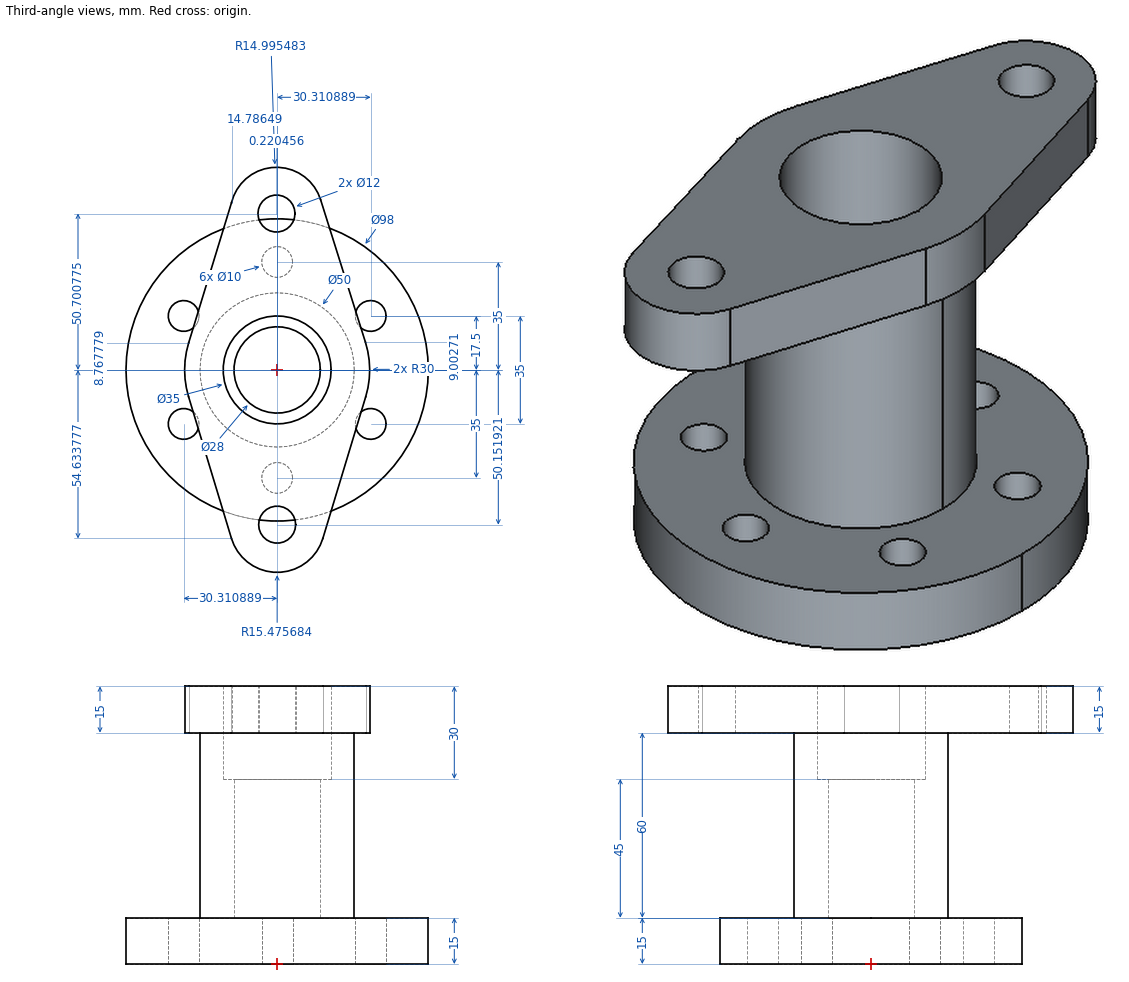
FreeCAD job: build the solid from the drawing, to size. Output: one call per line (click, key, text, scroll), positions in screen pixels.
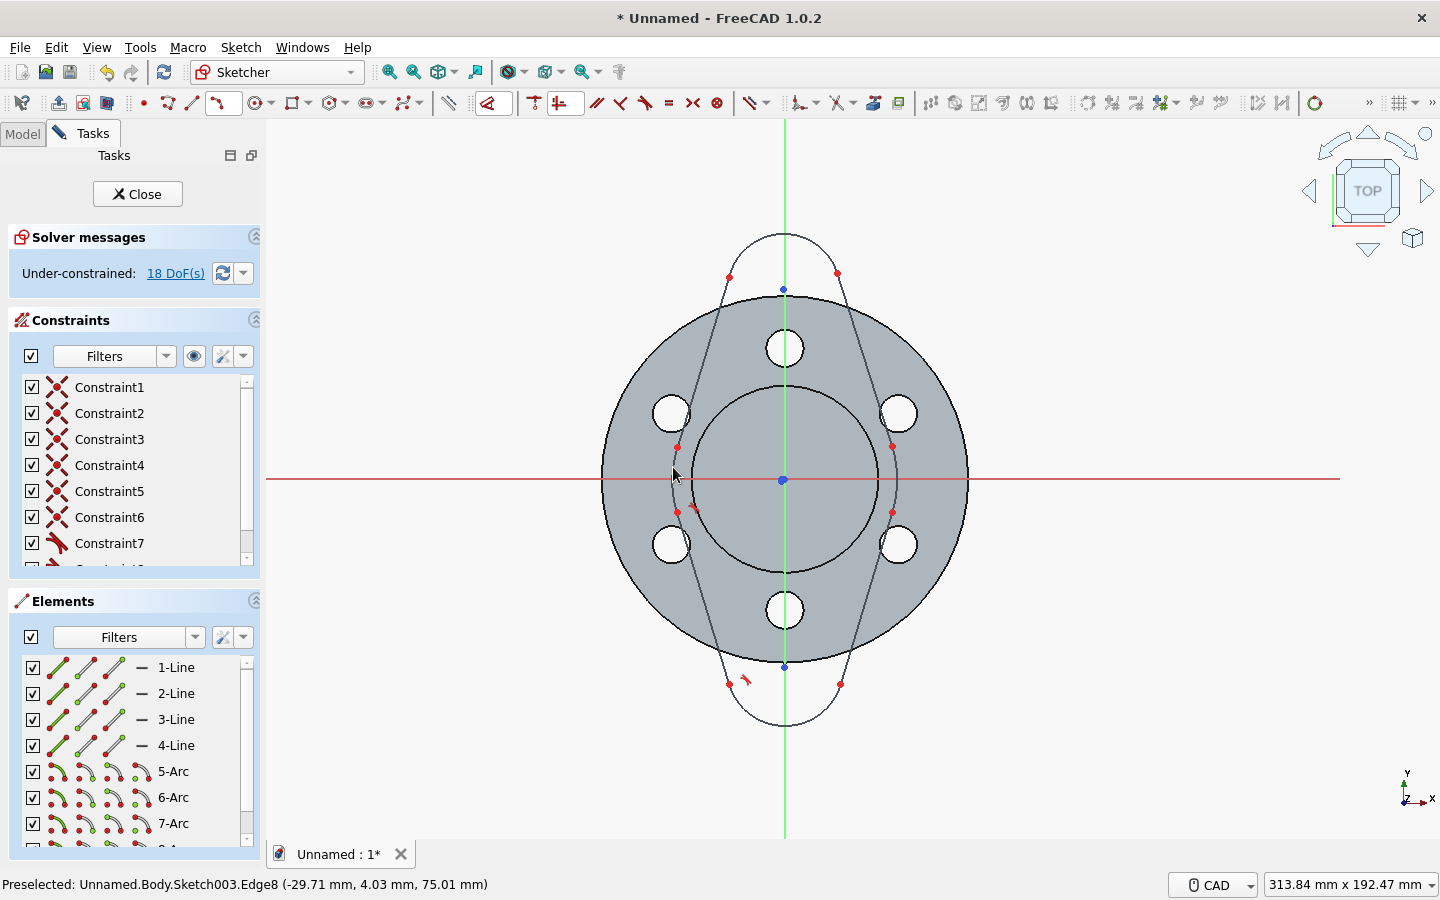
click(856, 633)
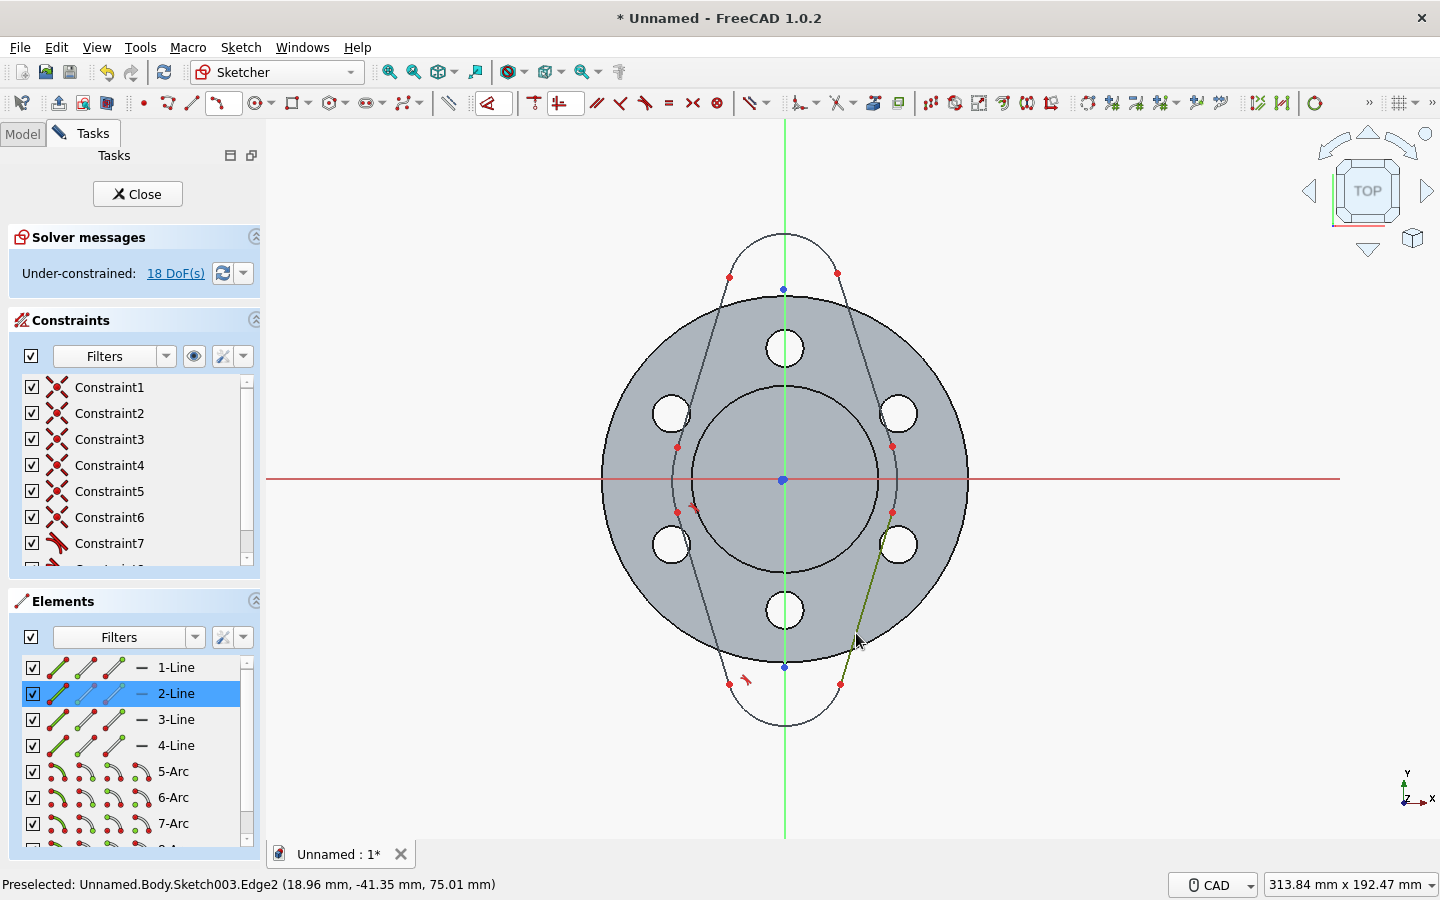
click(757, 719)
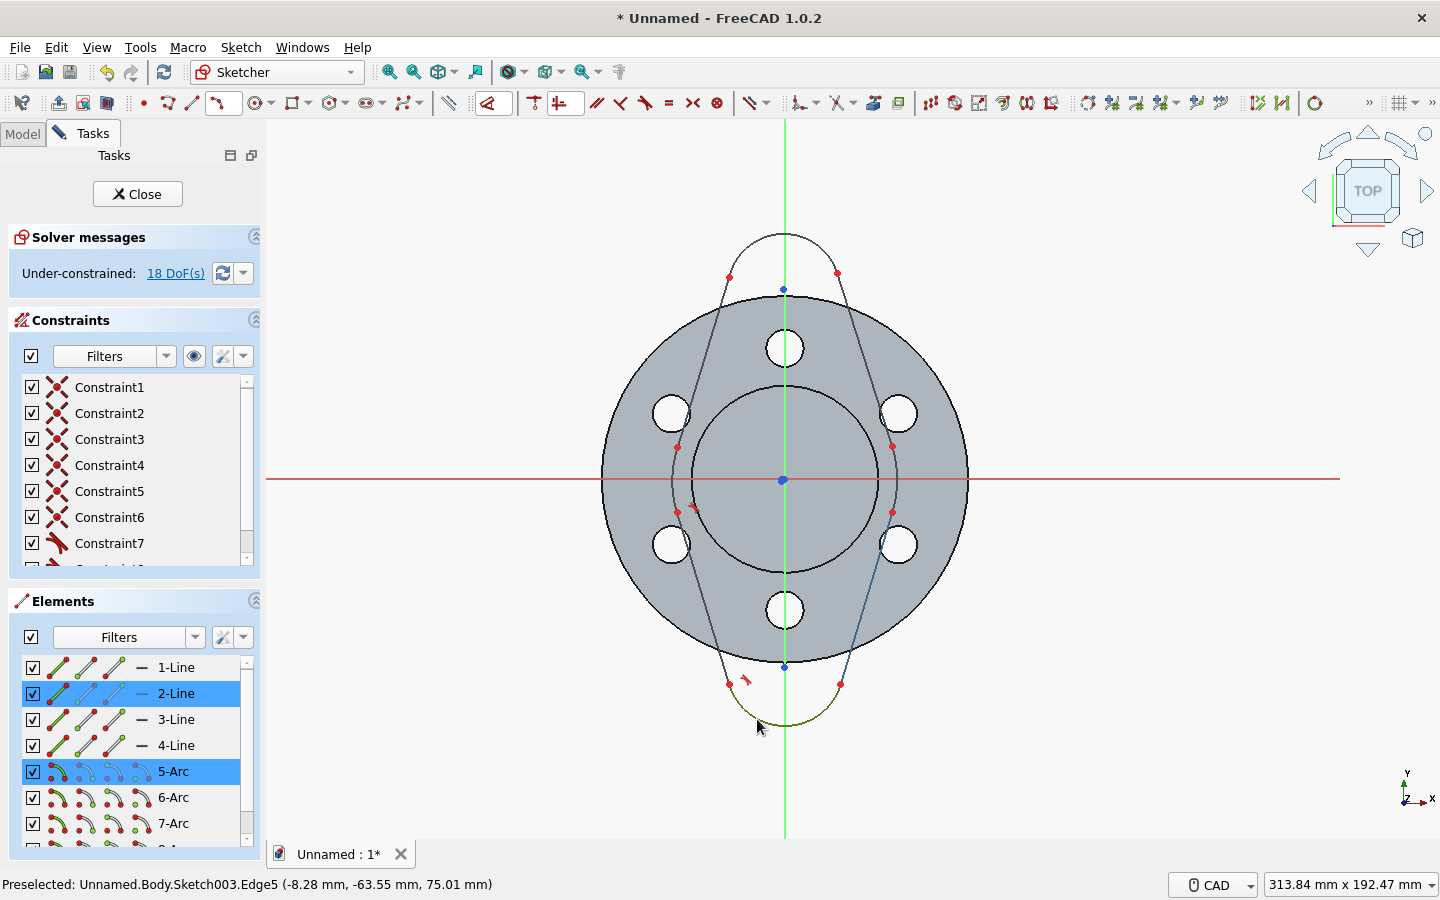
click(646, 104)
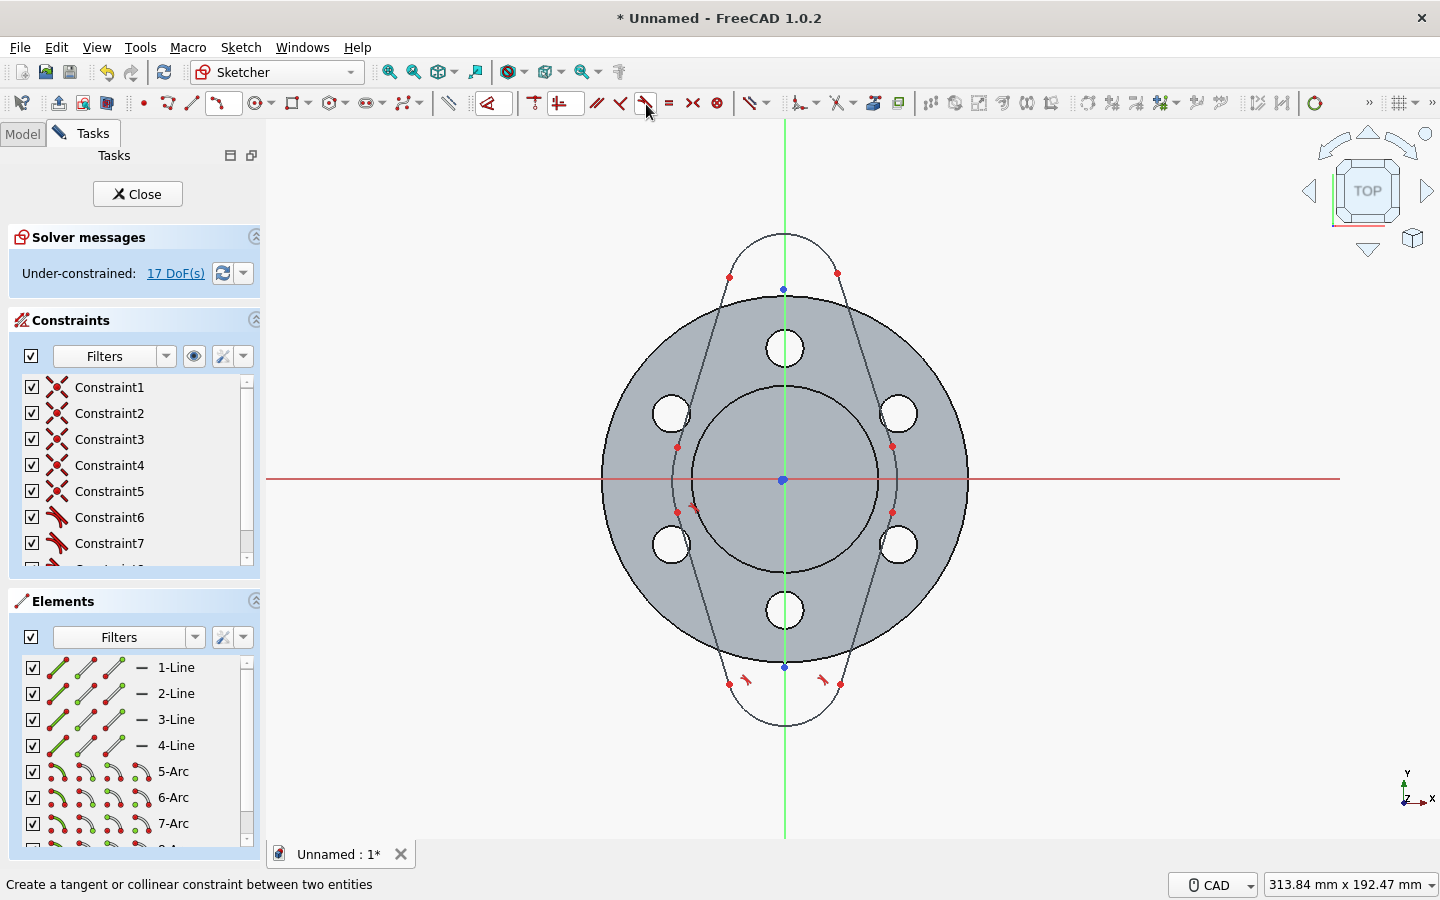
click(856, 633)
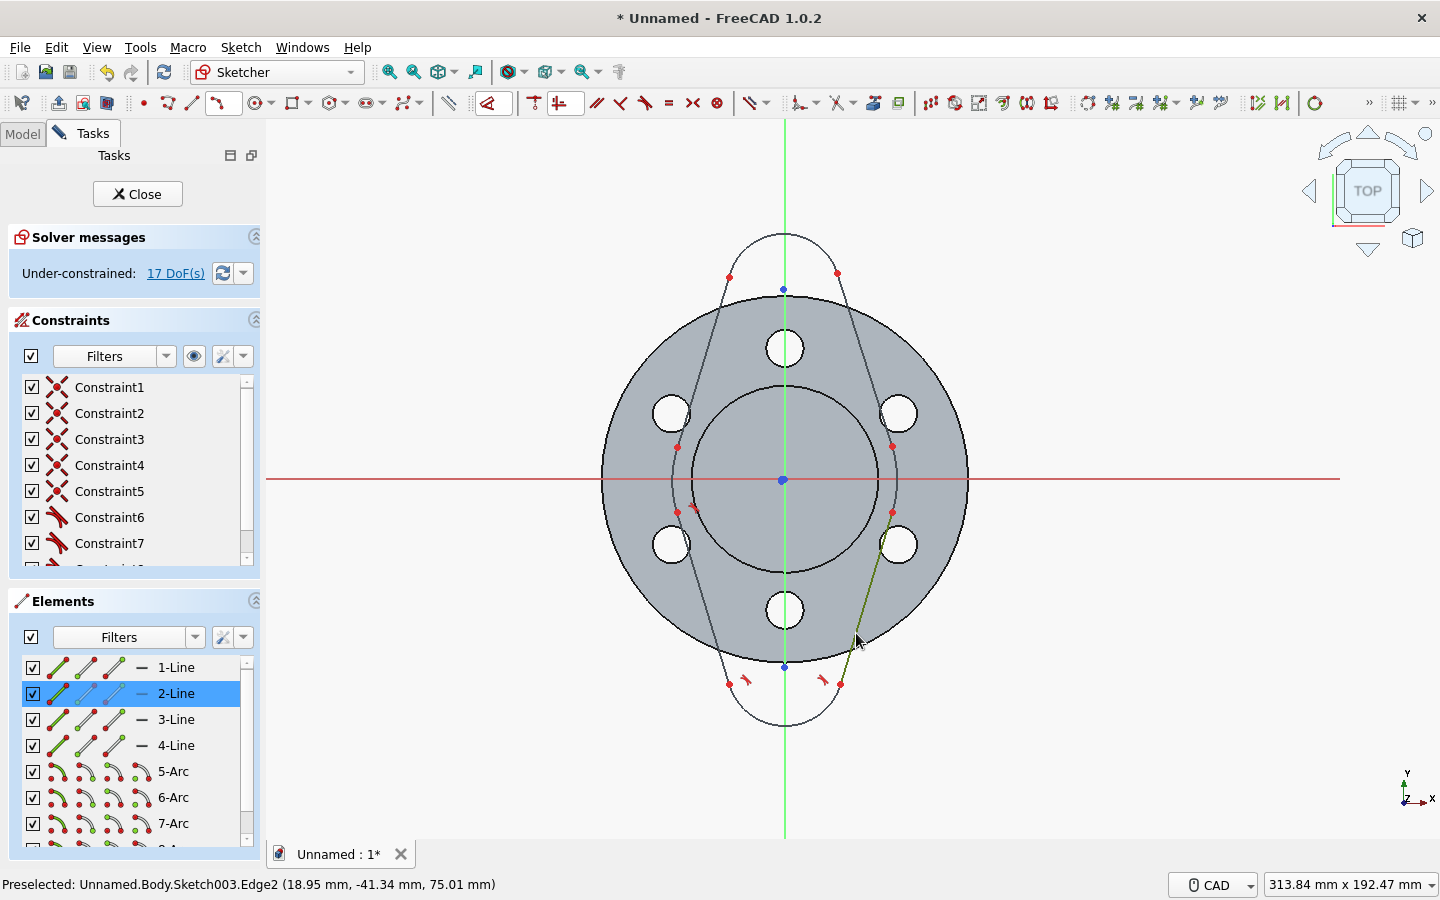
click(896, 493)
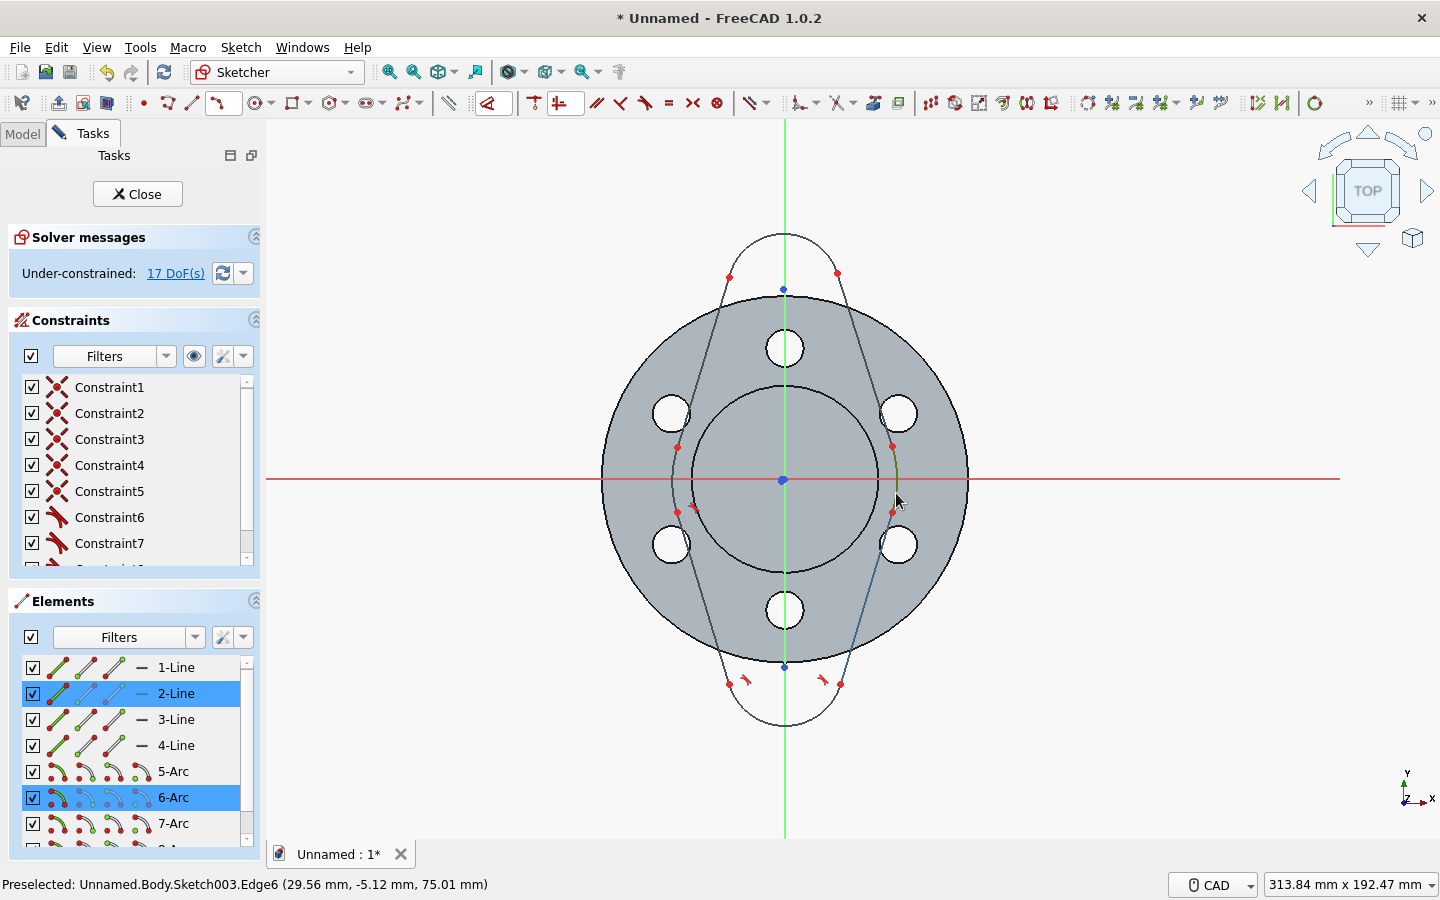
click(646, 104)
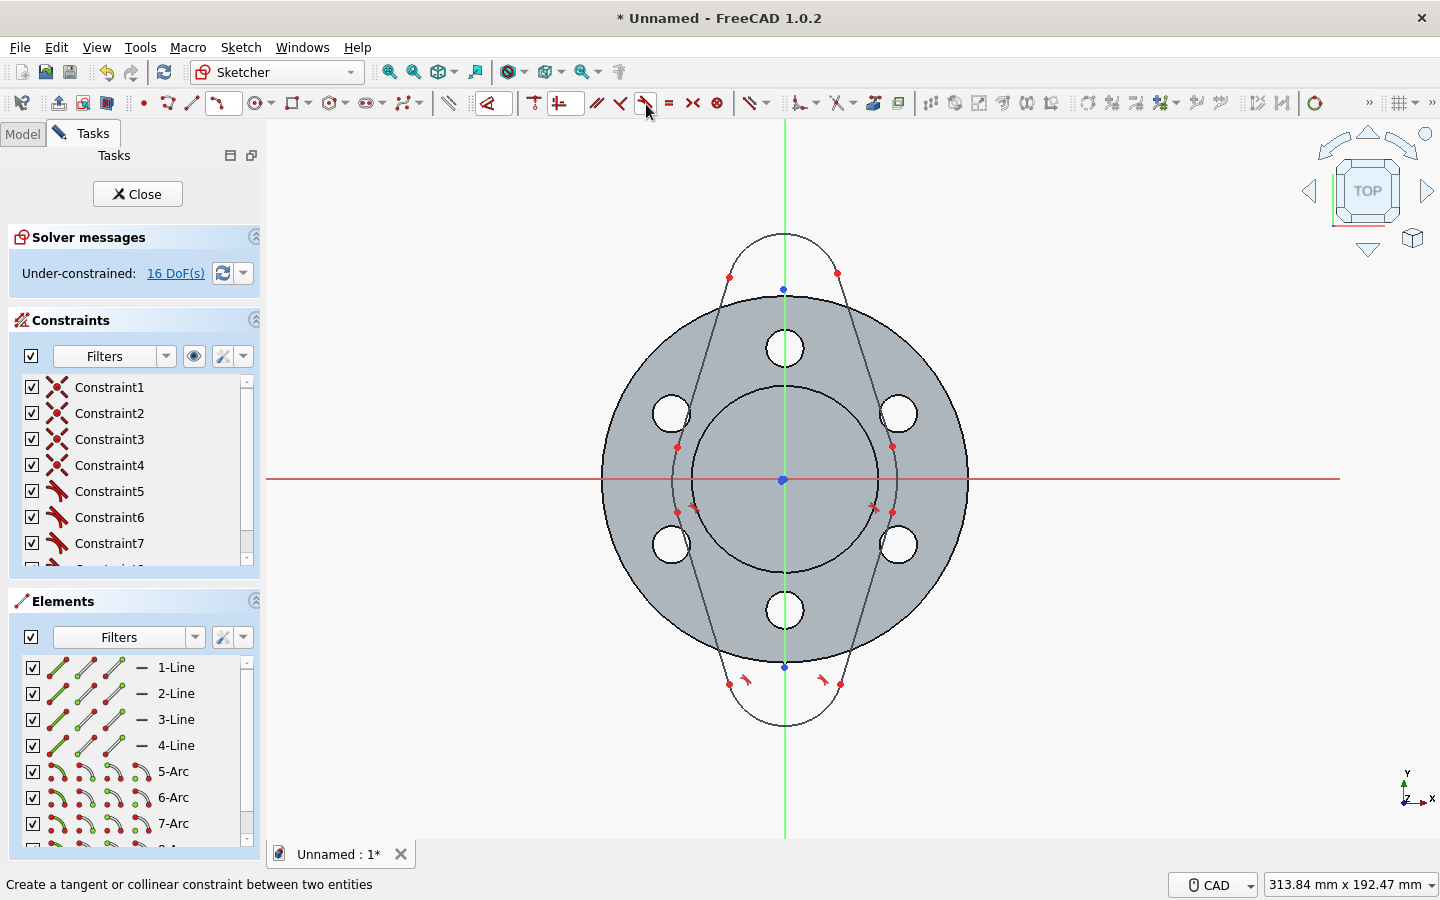
click(876, 395)